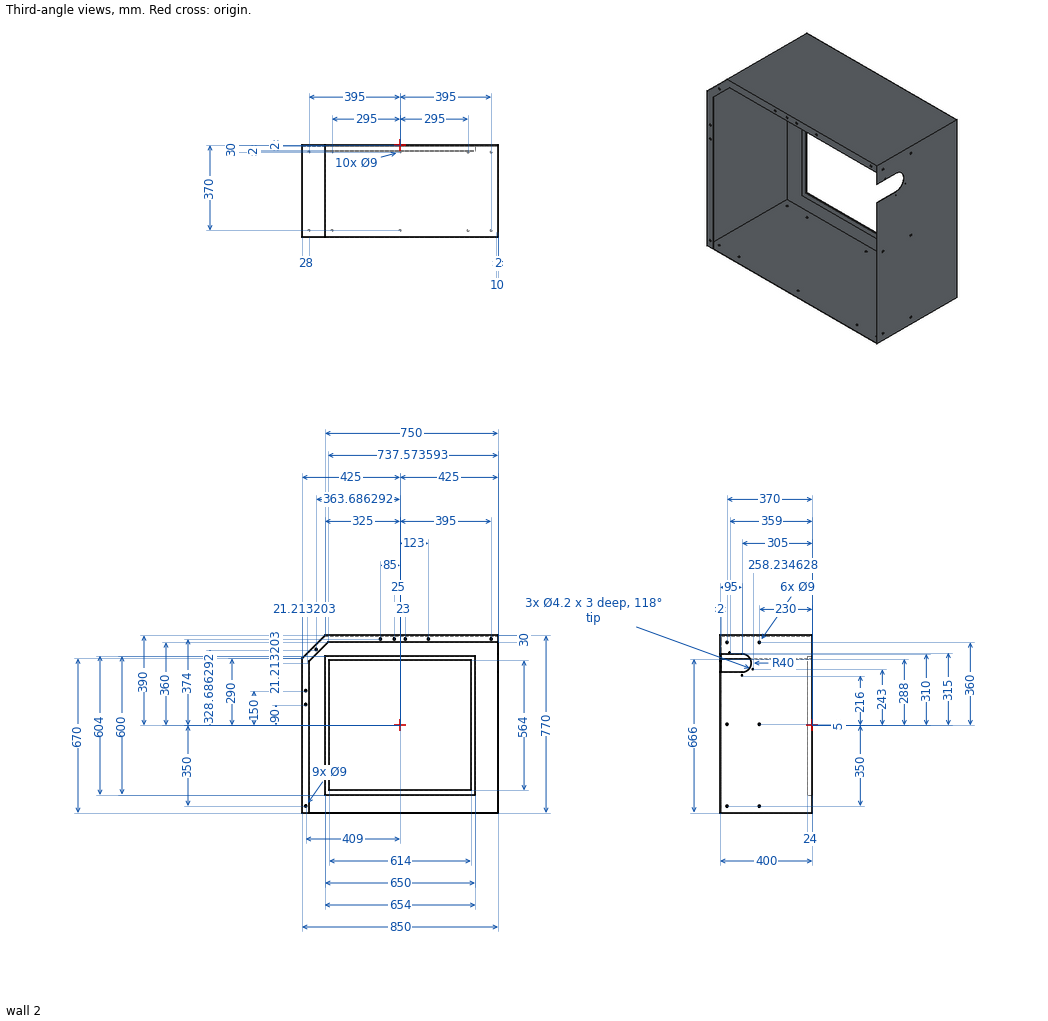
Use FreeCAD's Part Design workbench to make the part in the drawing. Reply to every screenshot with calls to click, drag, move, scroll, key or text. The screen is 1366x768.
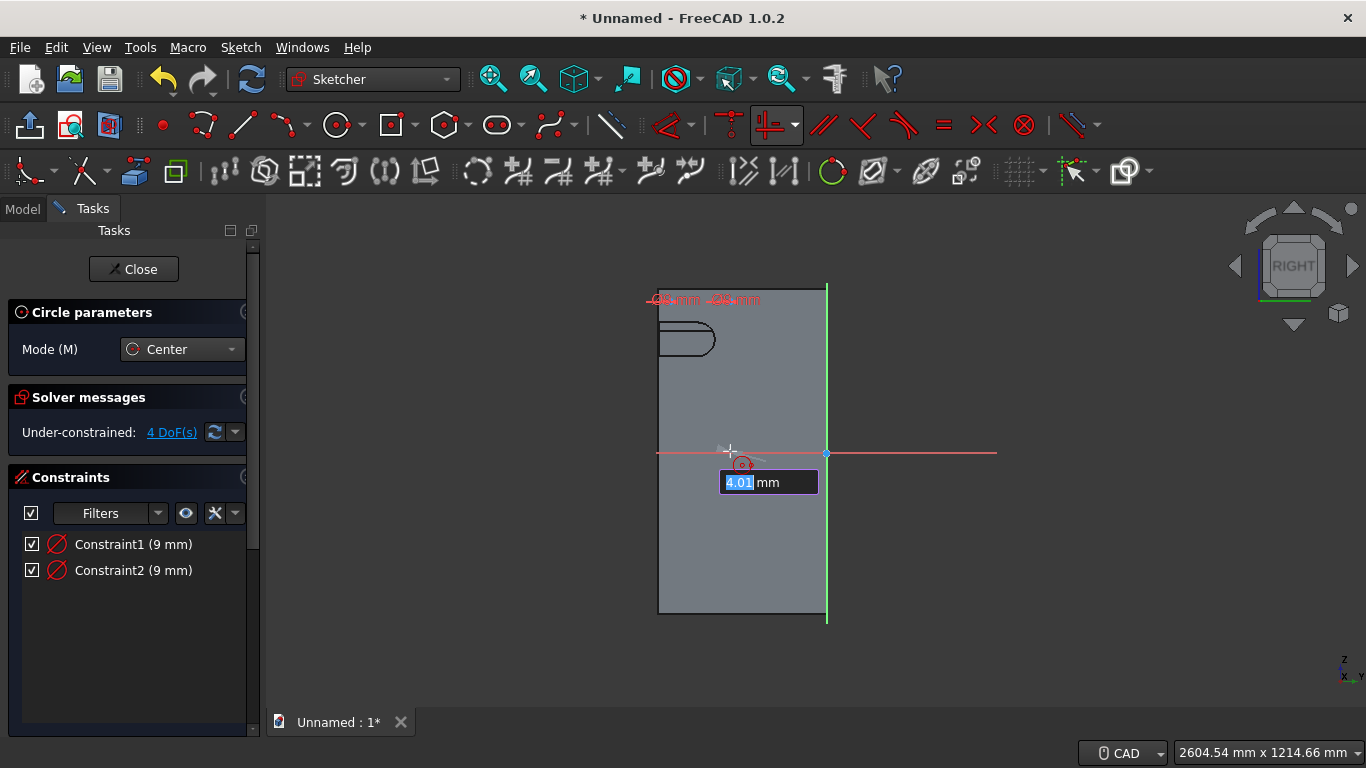
scroll(731, 450, up, 8)
move(729, 448)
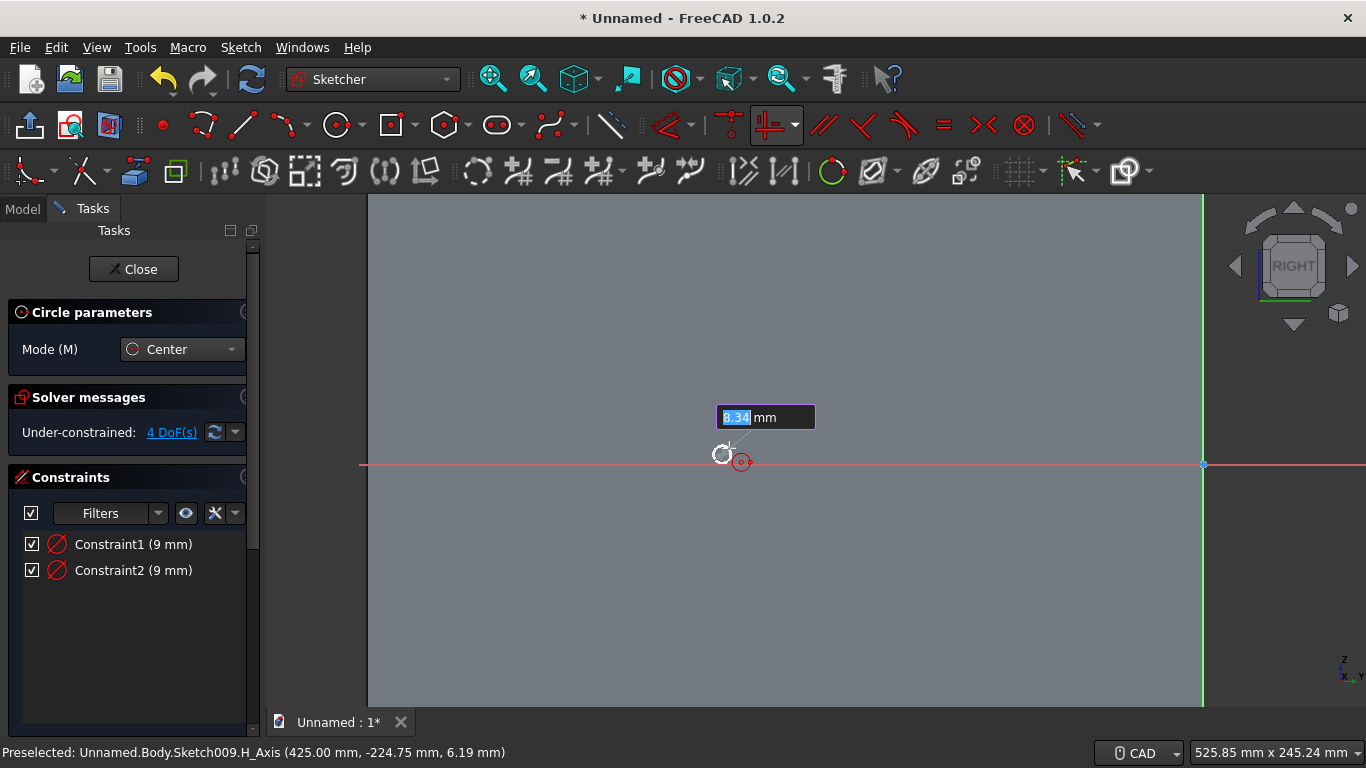
text(9)
key(Return)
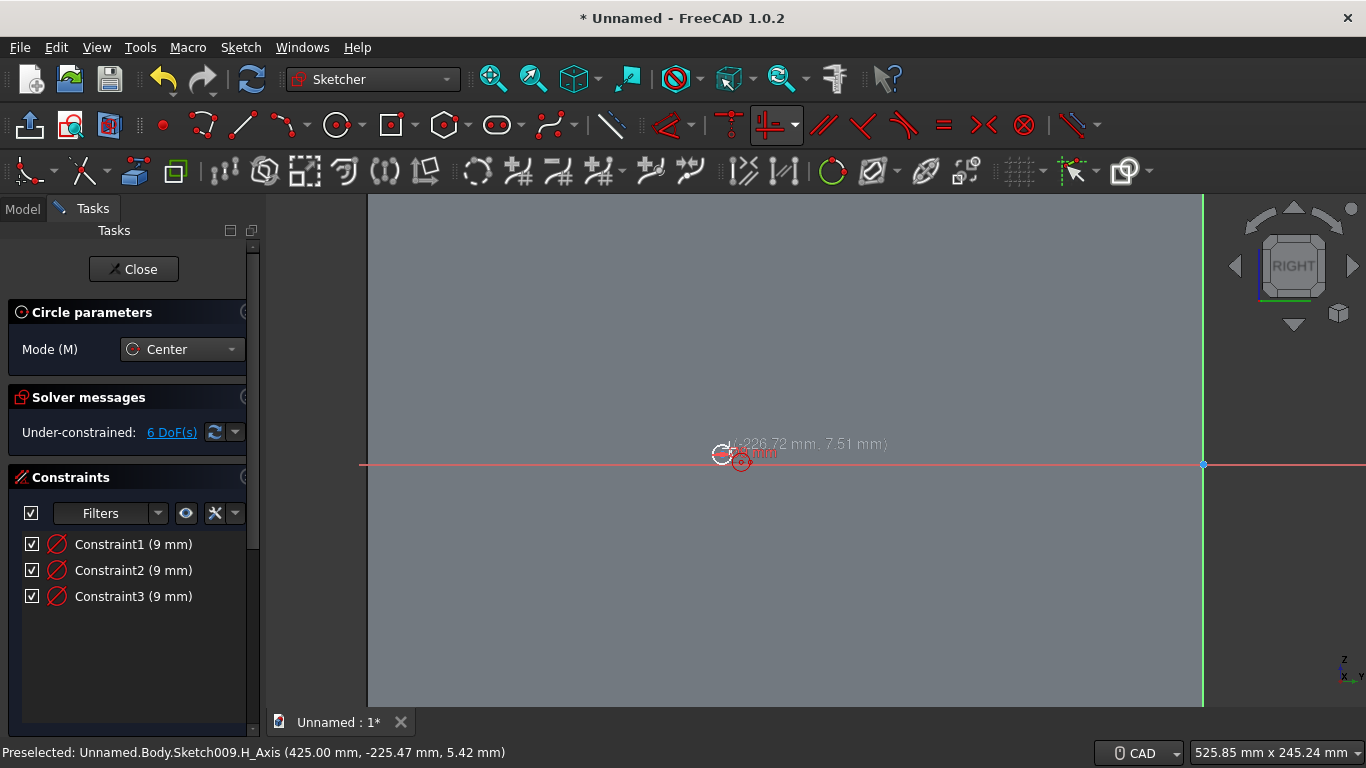
scroll(429, 454, up, 5)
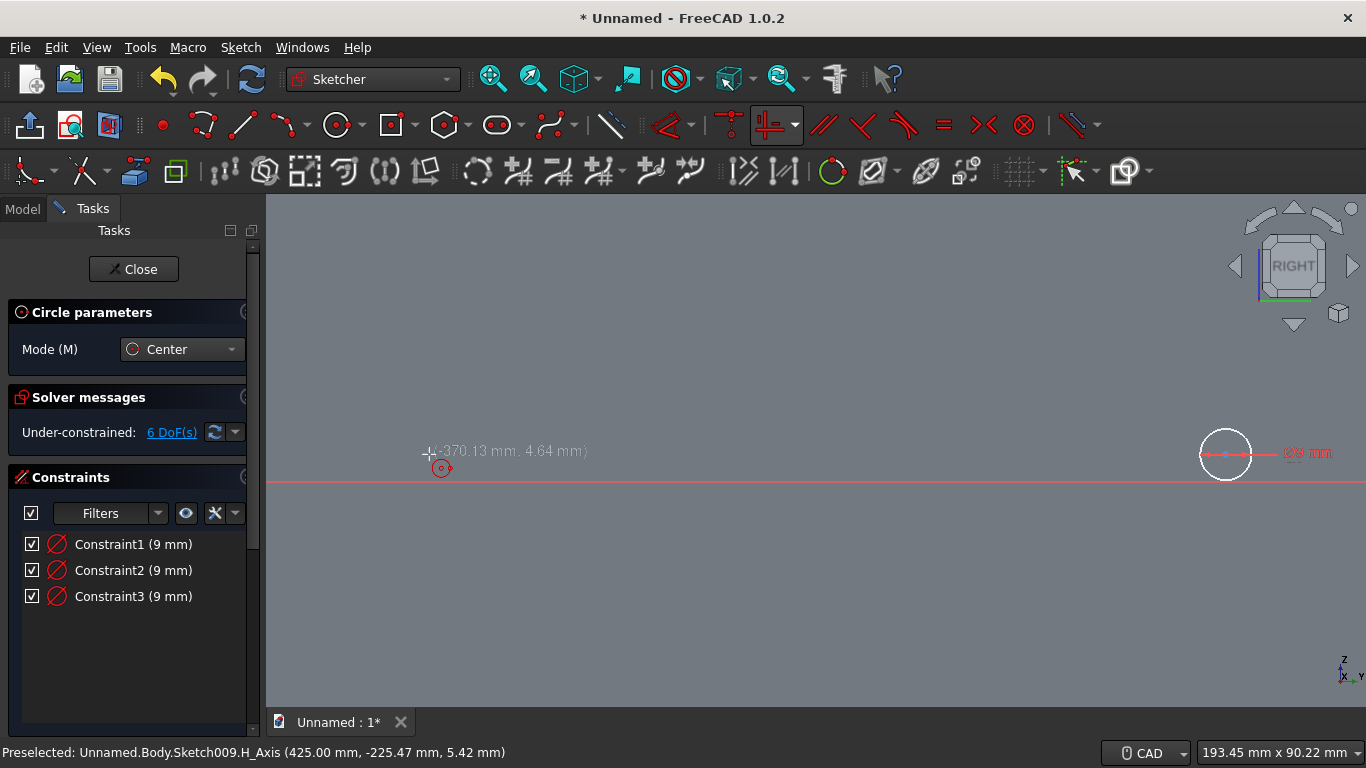
click(429, 454)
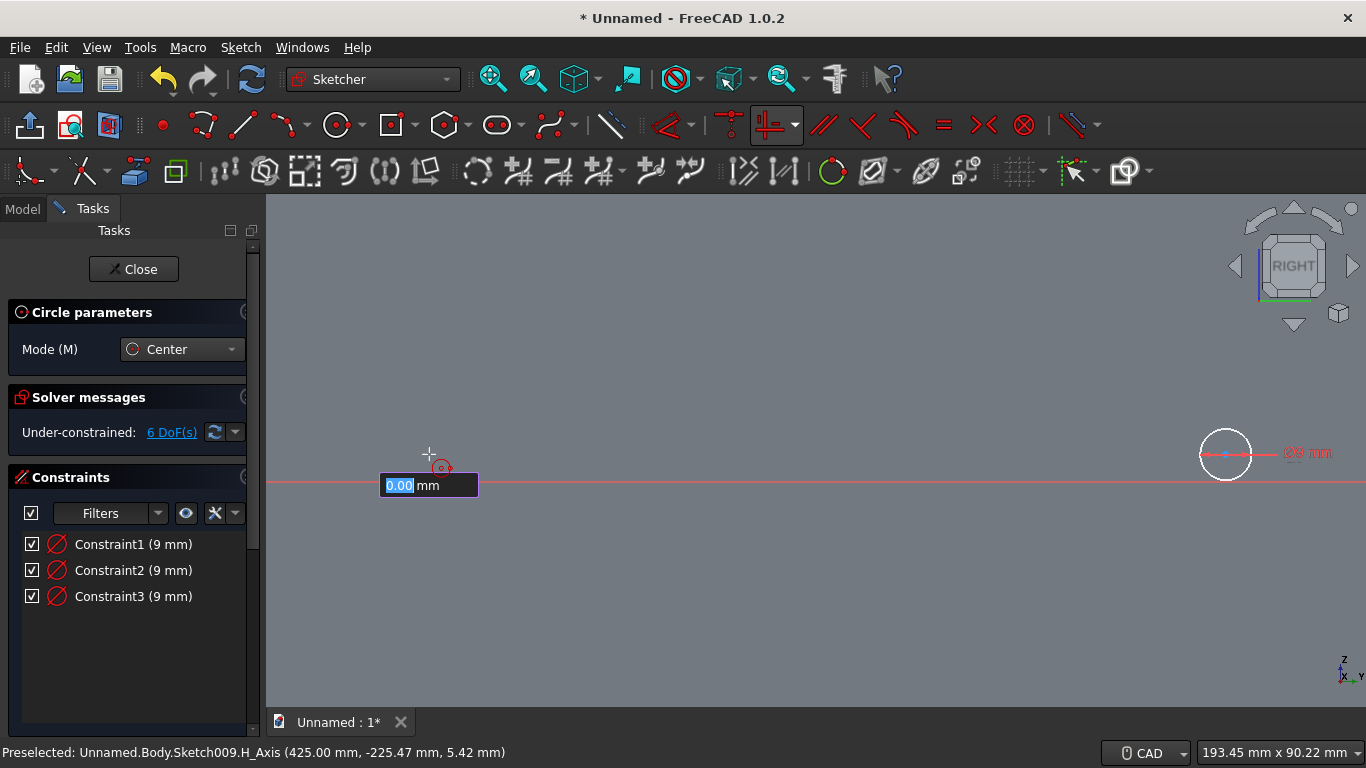
scroll(690, 450, down, 13)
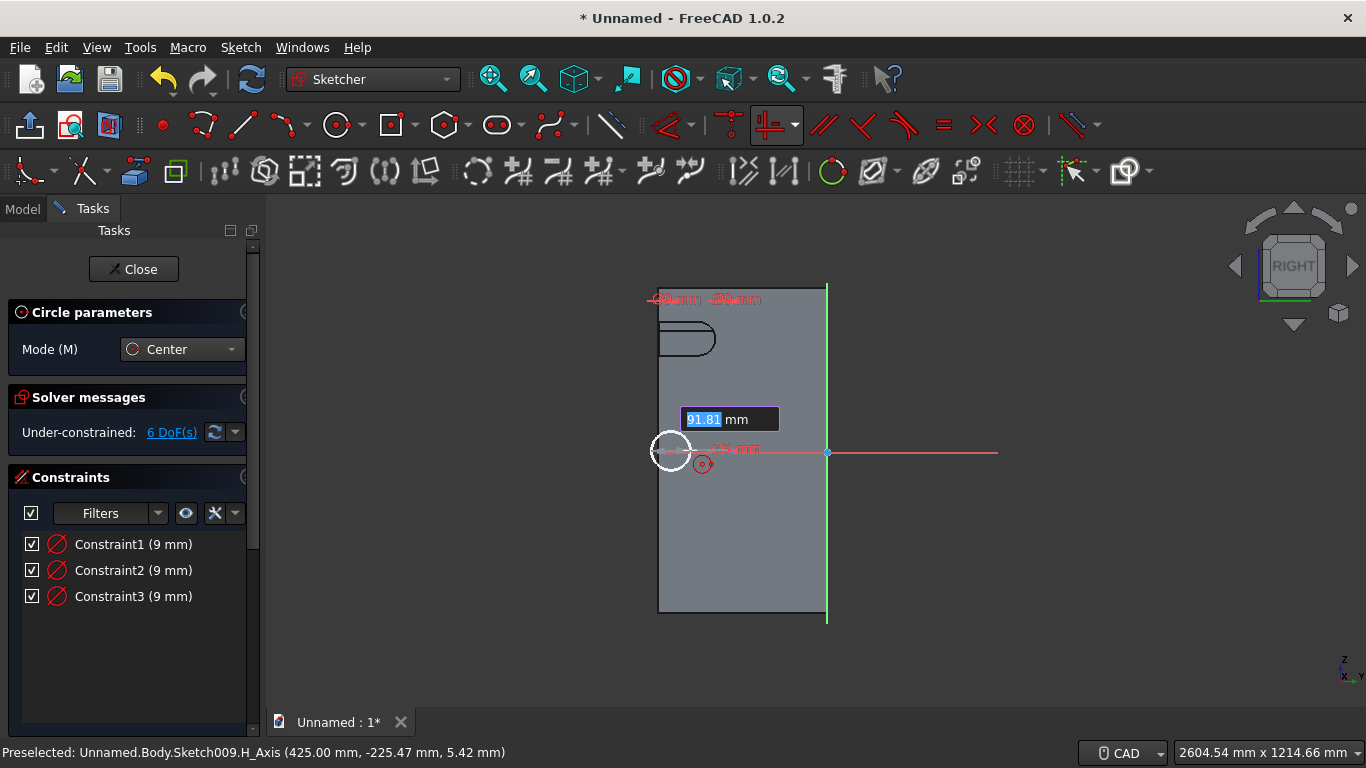
scroll(672, 449, up, 8)
move(672, 449)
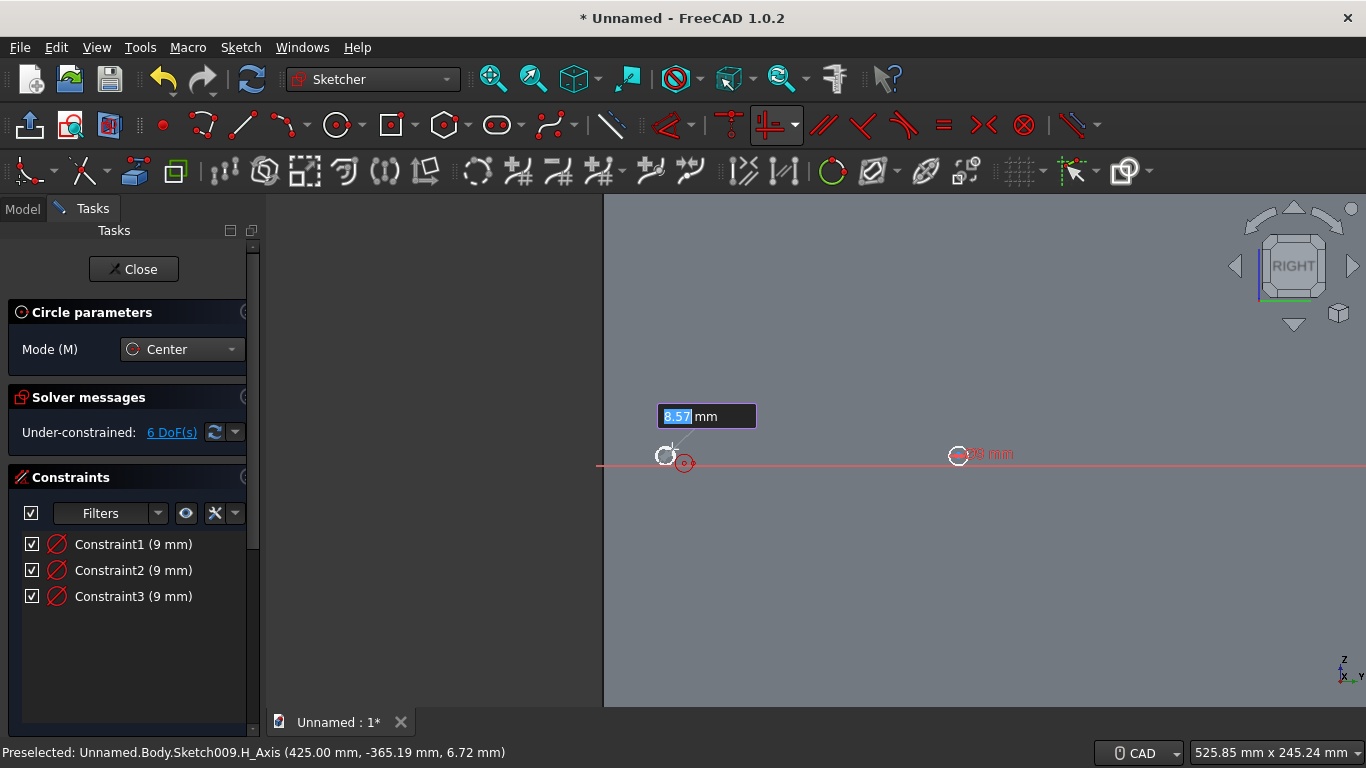
text(9)
key(Return)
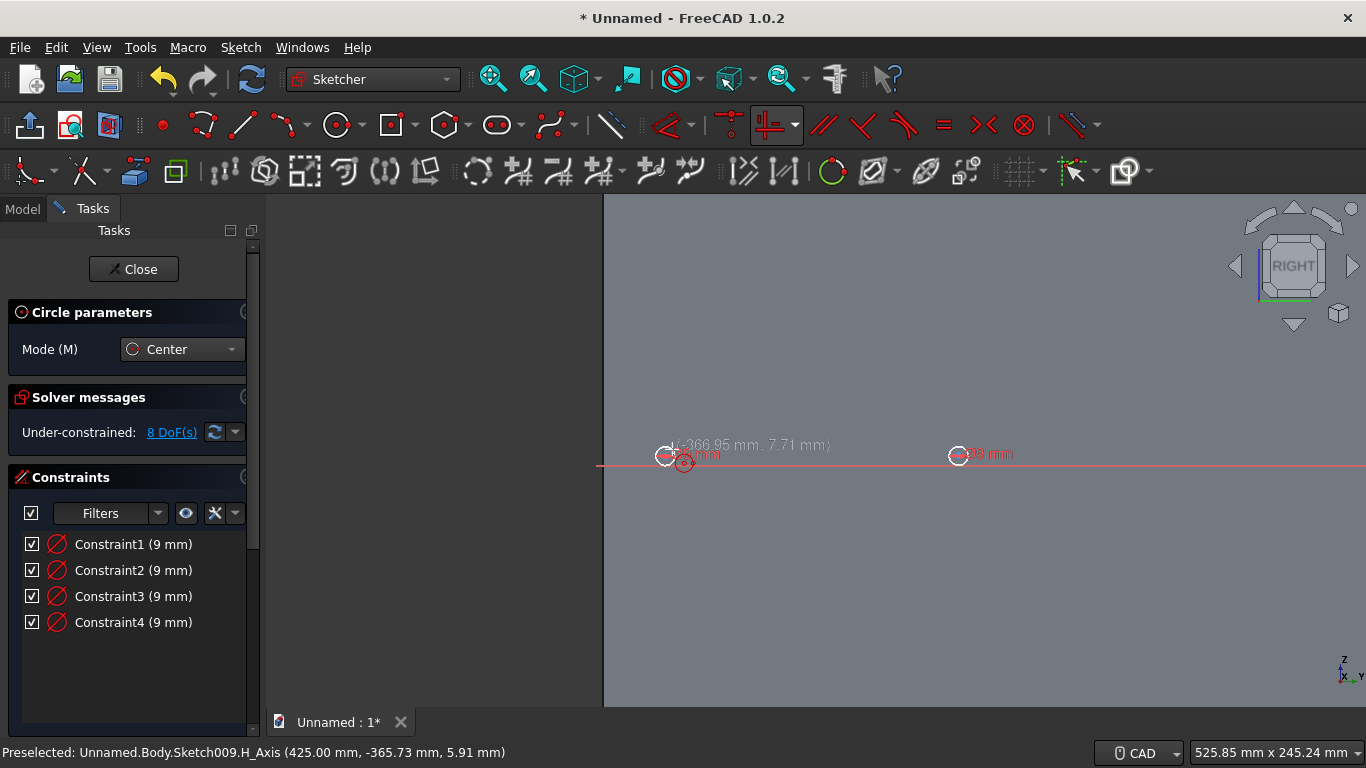
scroll(672, 449, down, 8)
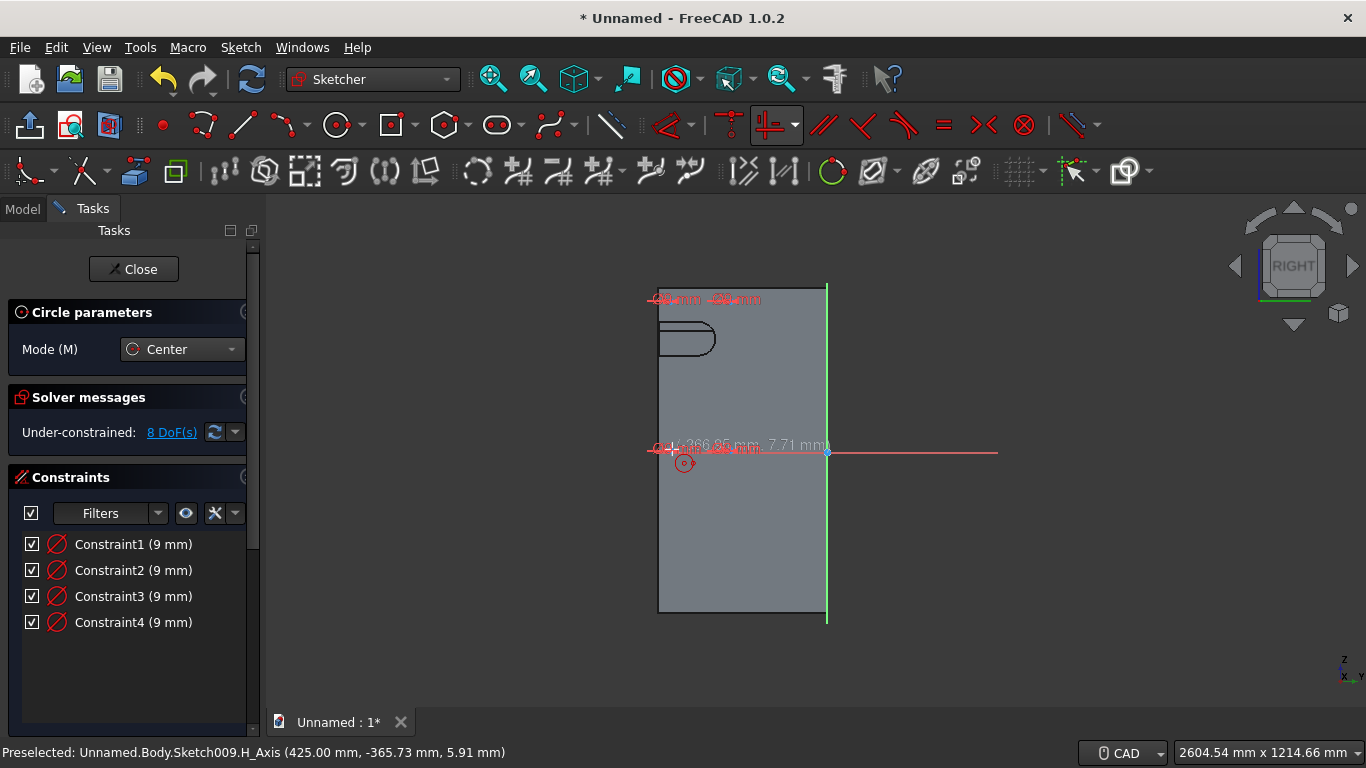
scroll(671, 601, up, 13)